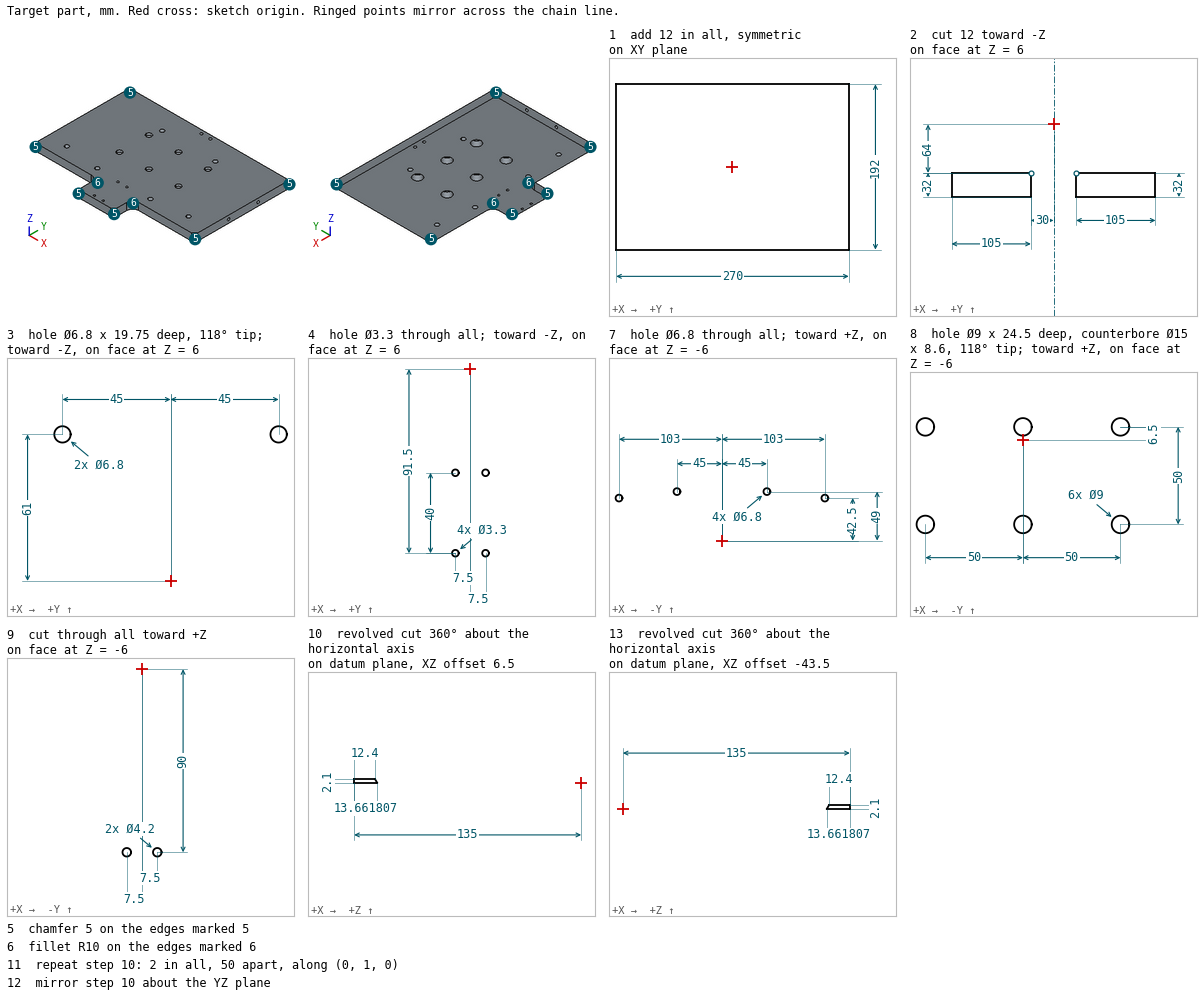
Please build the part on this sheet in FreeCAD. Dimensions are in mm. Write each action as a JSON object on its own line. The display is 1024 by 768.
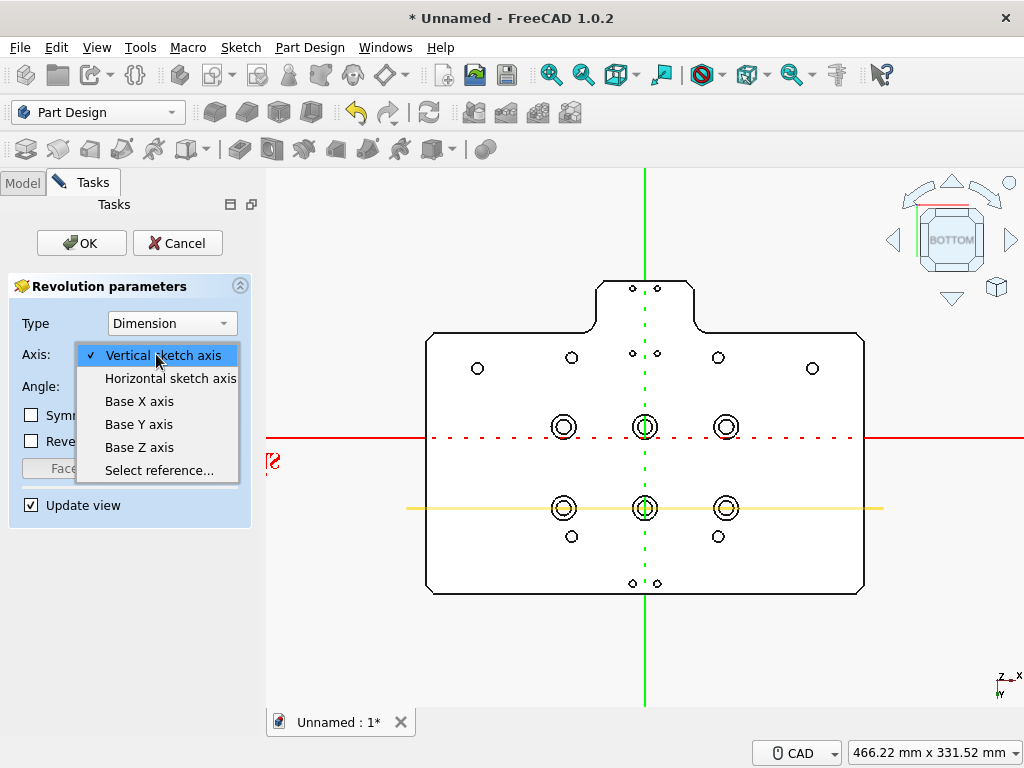
{"action": "left_click", "coordinate": [156, 378]}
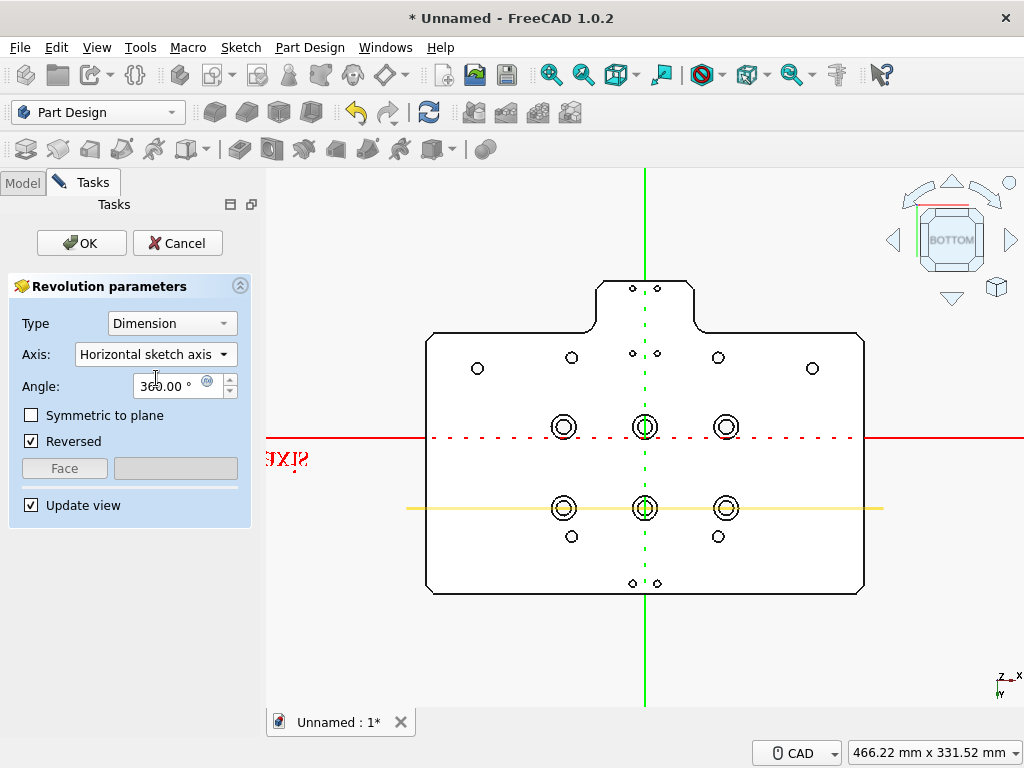
{"action": "left_click", "coordinate": [82, 243]}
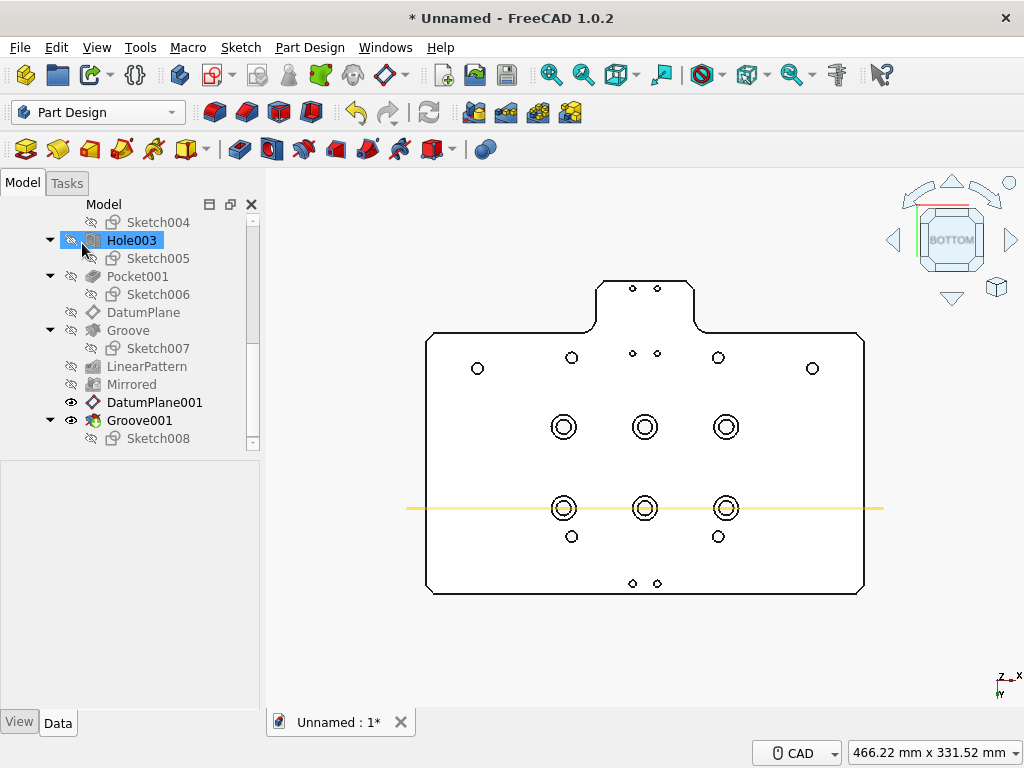
{"action": "left_click", "coordinate": [116, 402]}
{"action": "key", "text": "space"}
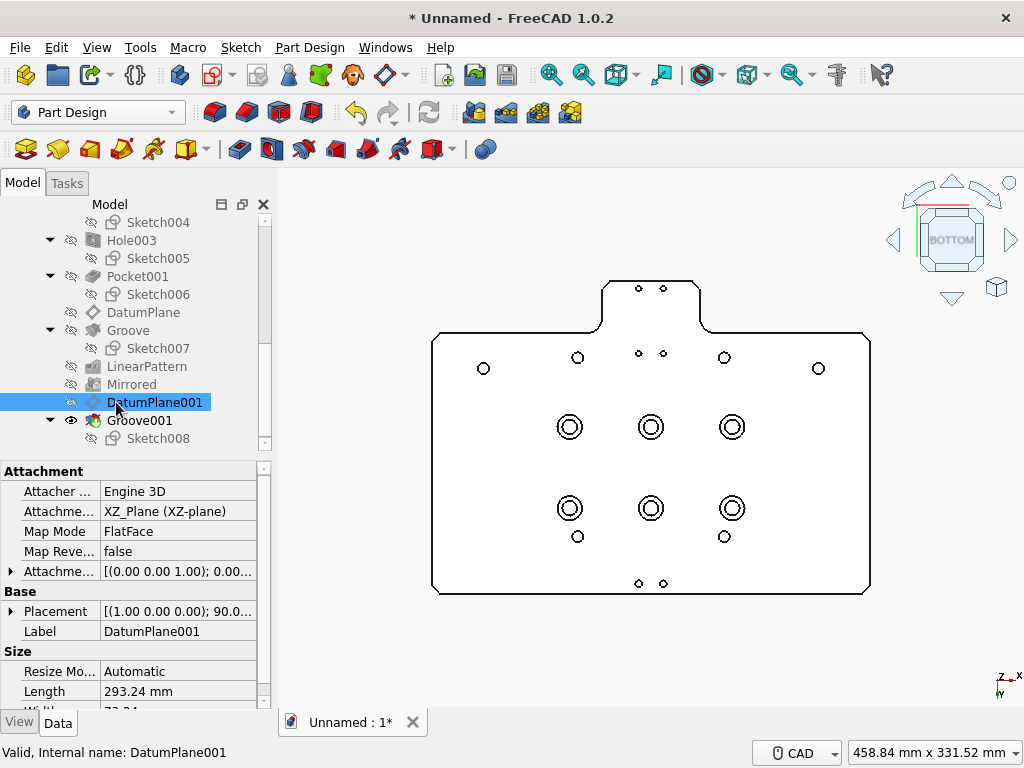
{"action": "key", "text": "0"}